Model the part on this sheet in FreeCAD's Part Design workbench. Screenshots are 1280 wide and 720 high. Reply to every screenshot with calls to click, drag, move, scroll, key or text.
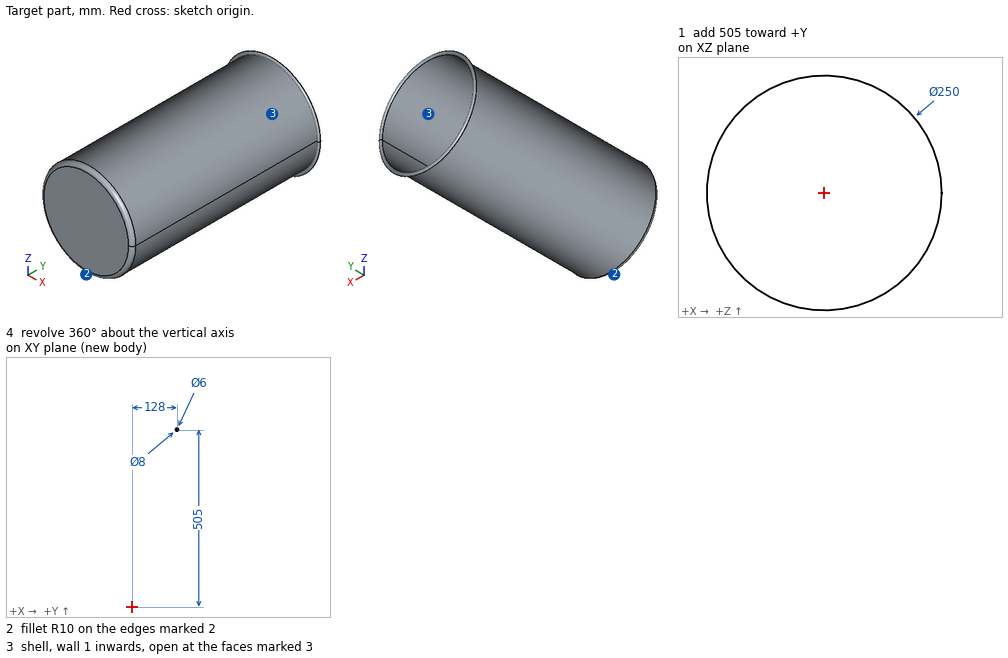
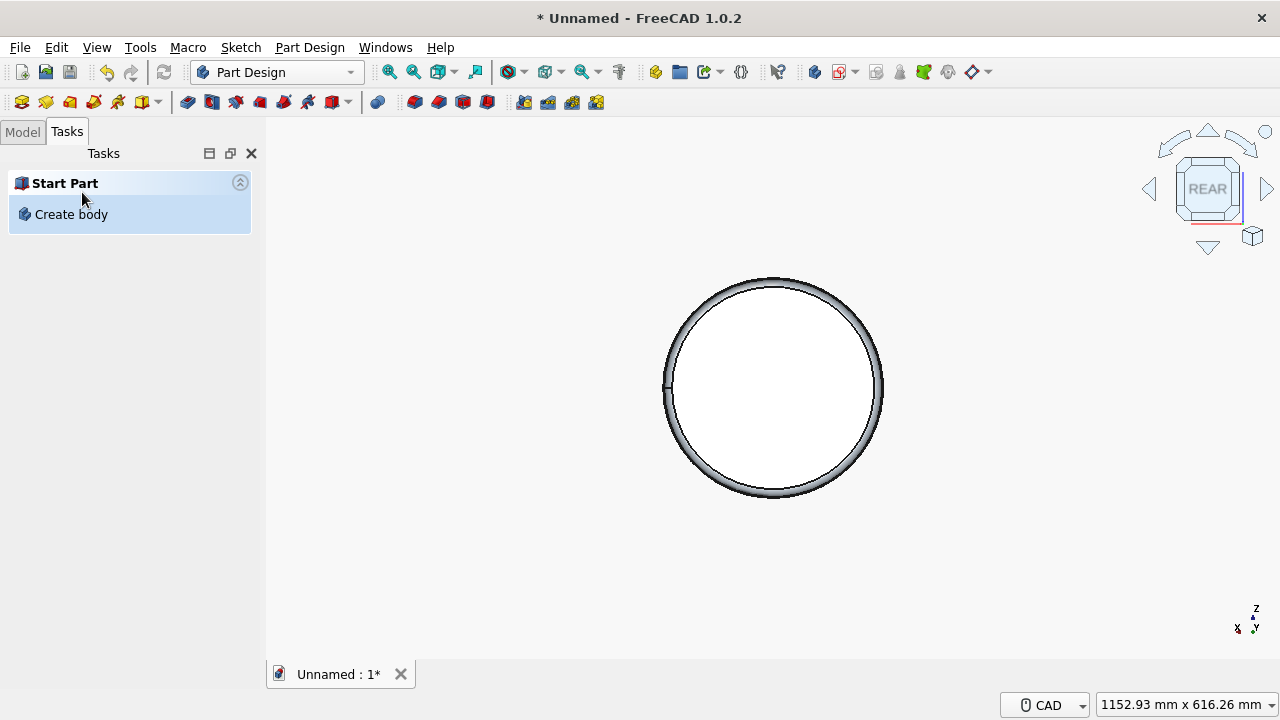
click(390, 72)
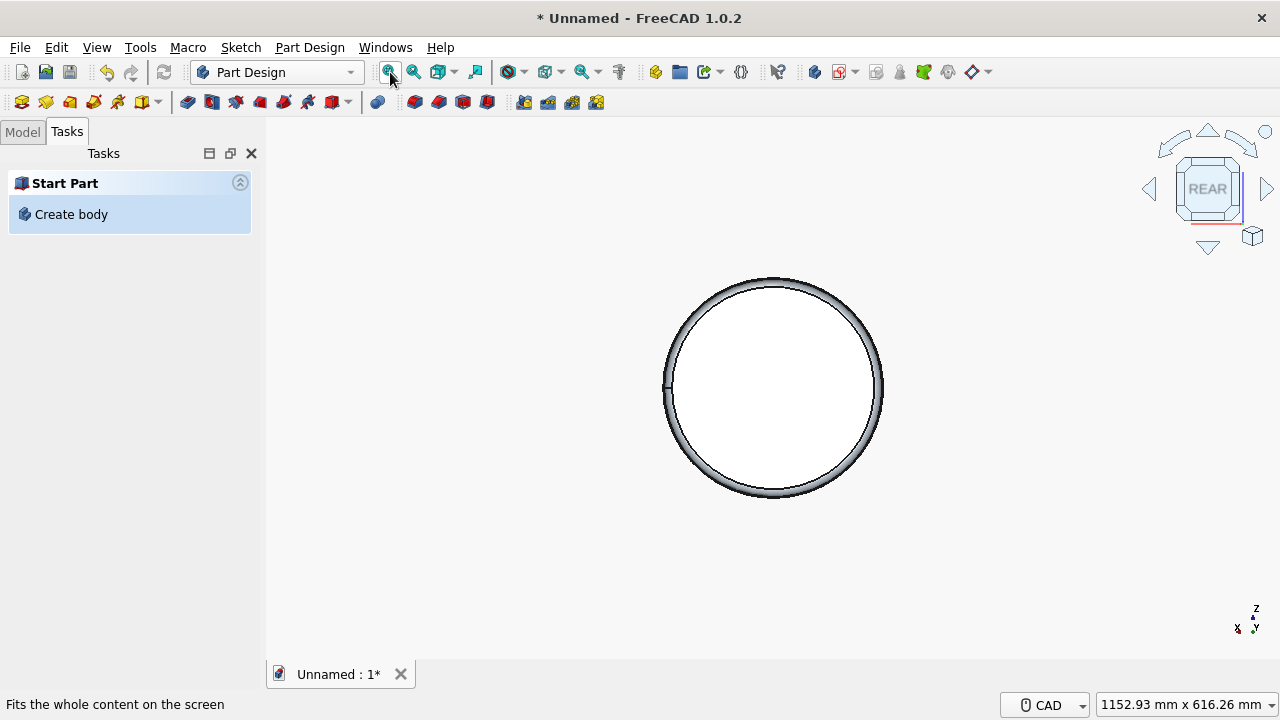
click(816, 72)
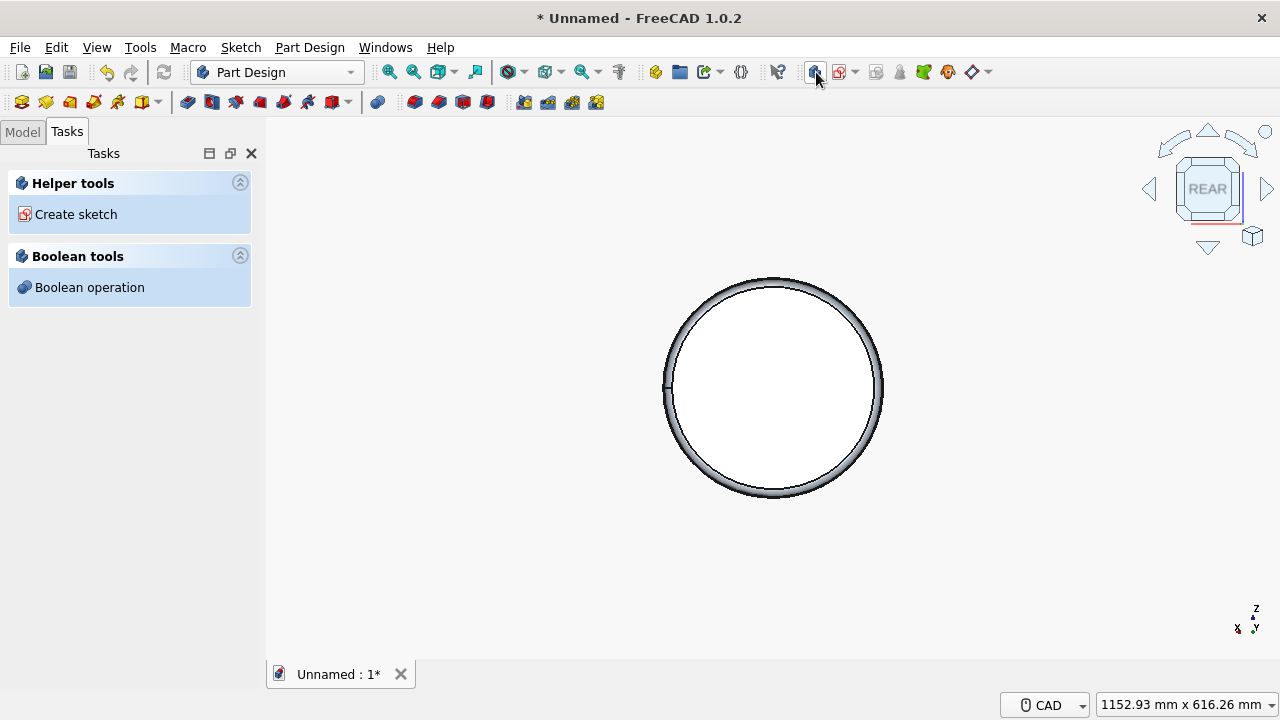
click(306, 619)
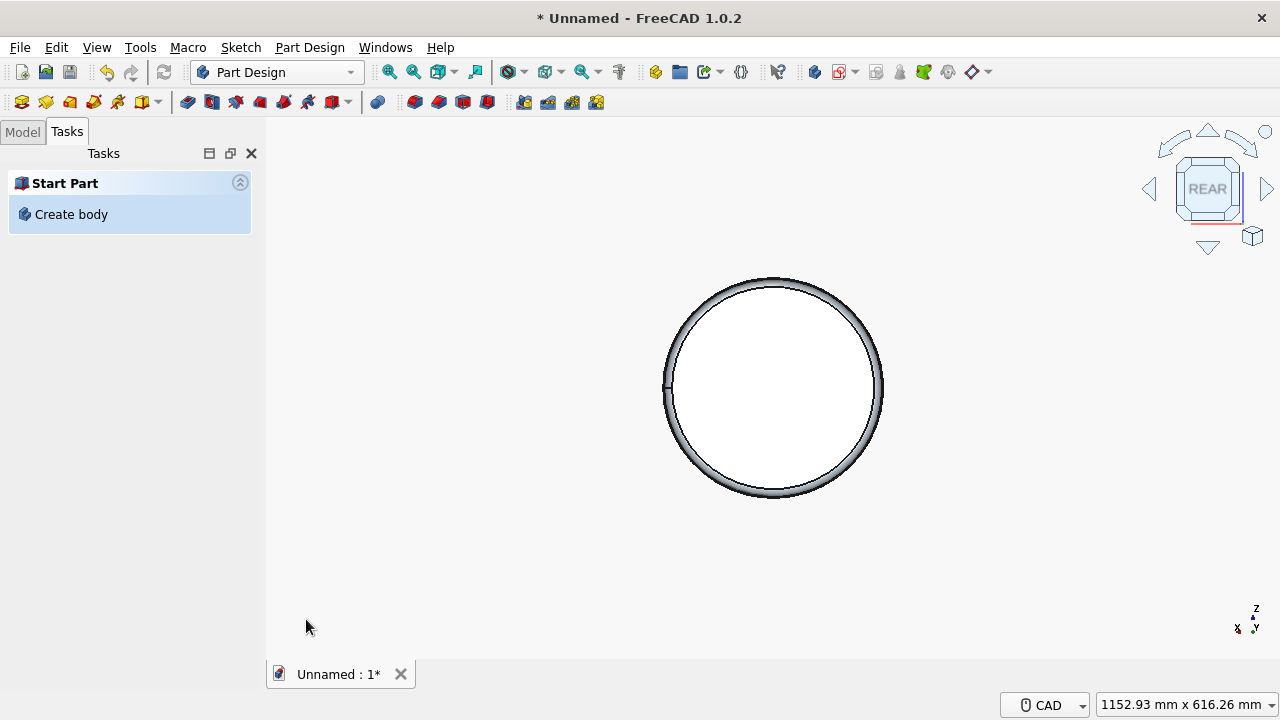
click(840, 72)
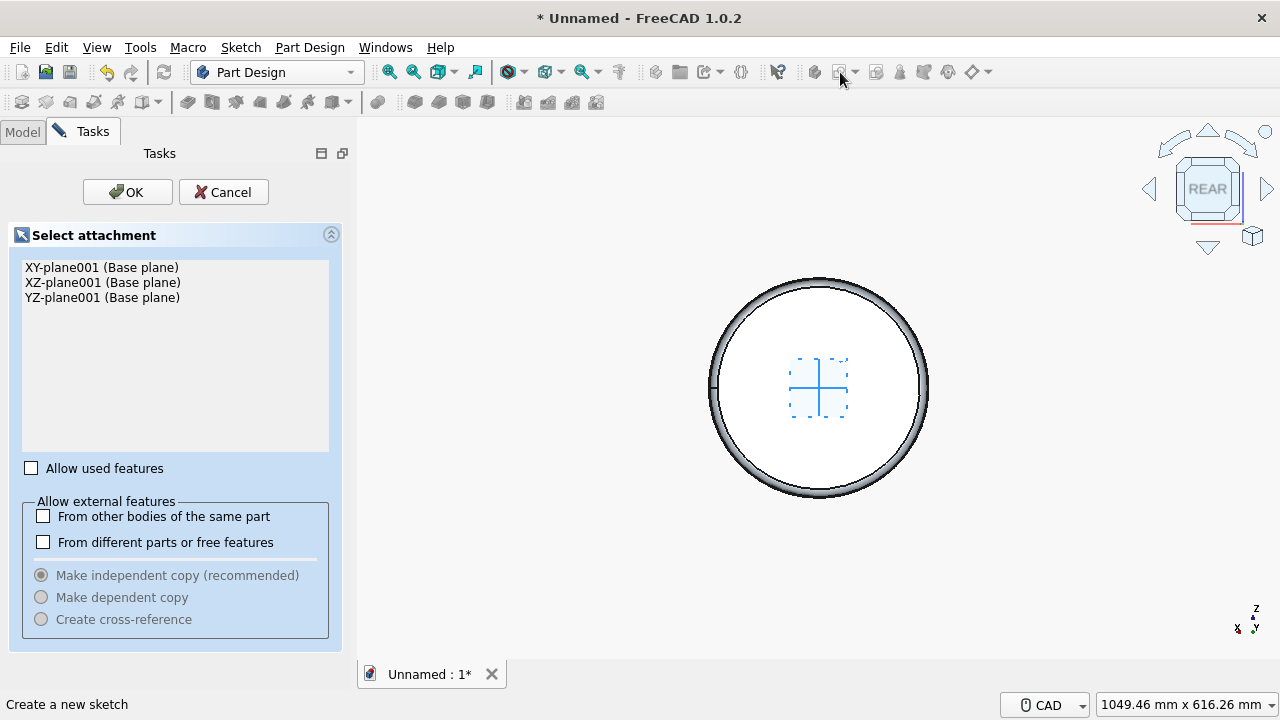
click(82, 268)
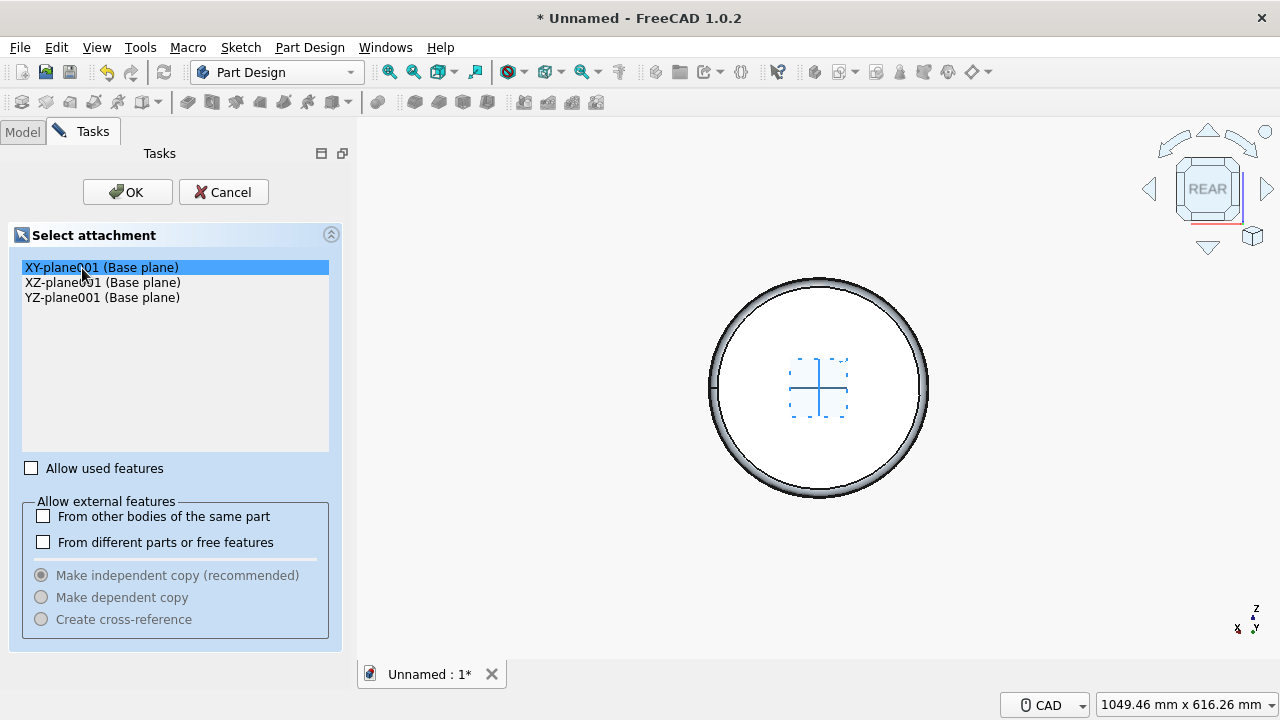
click(128, 192)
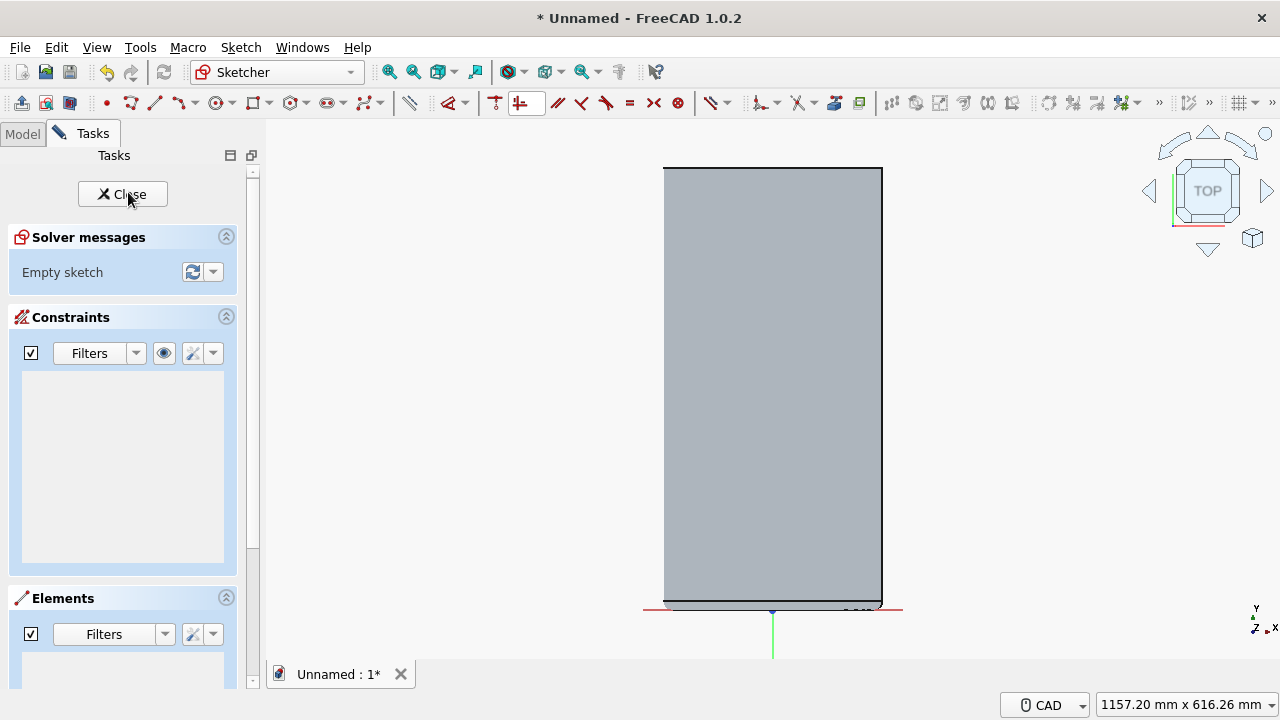
scroll(894, 156, up, 15)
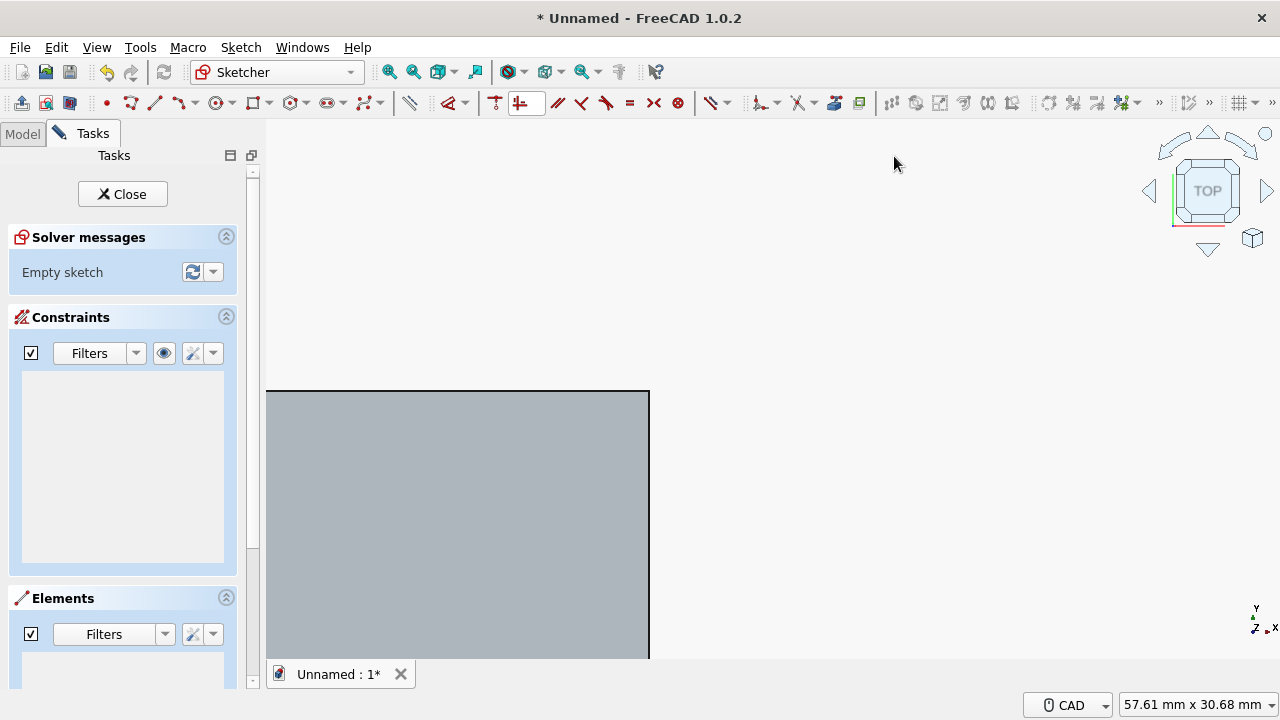
scroll(699, 392, up, 4)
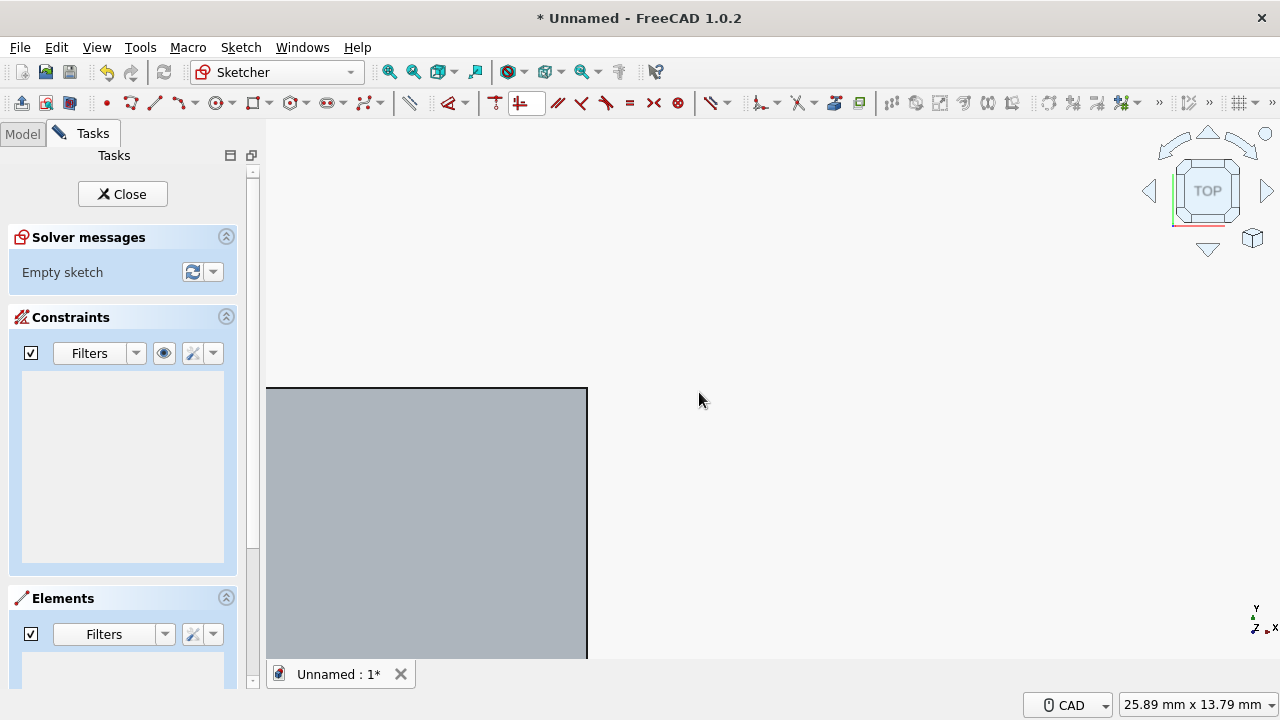
click(216, 104)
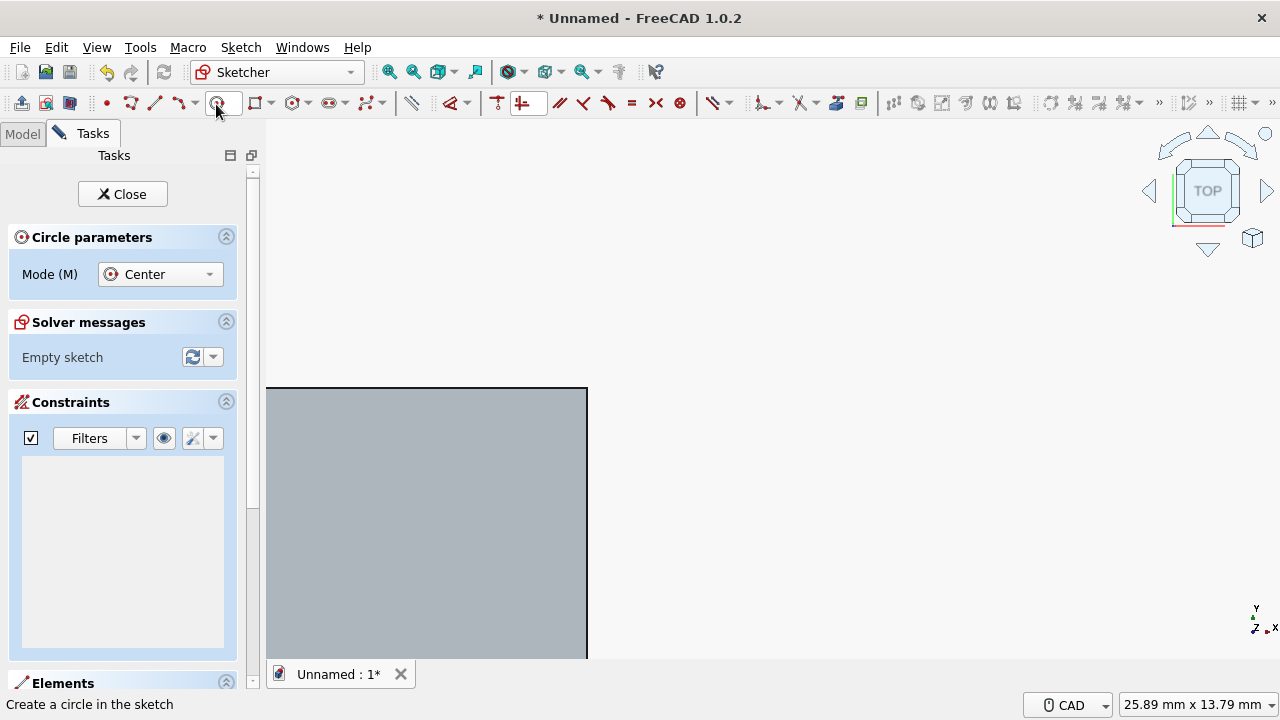
click(704, 388)
move(815, 277)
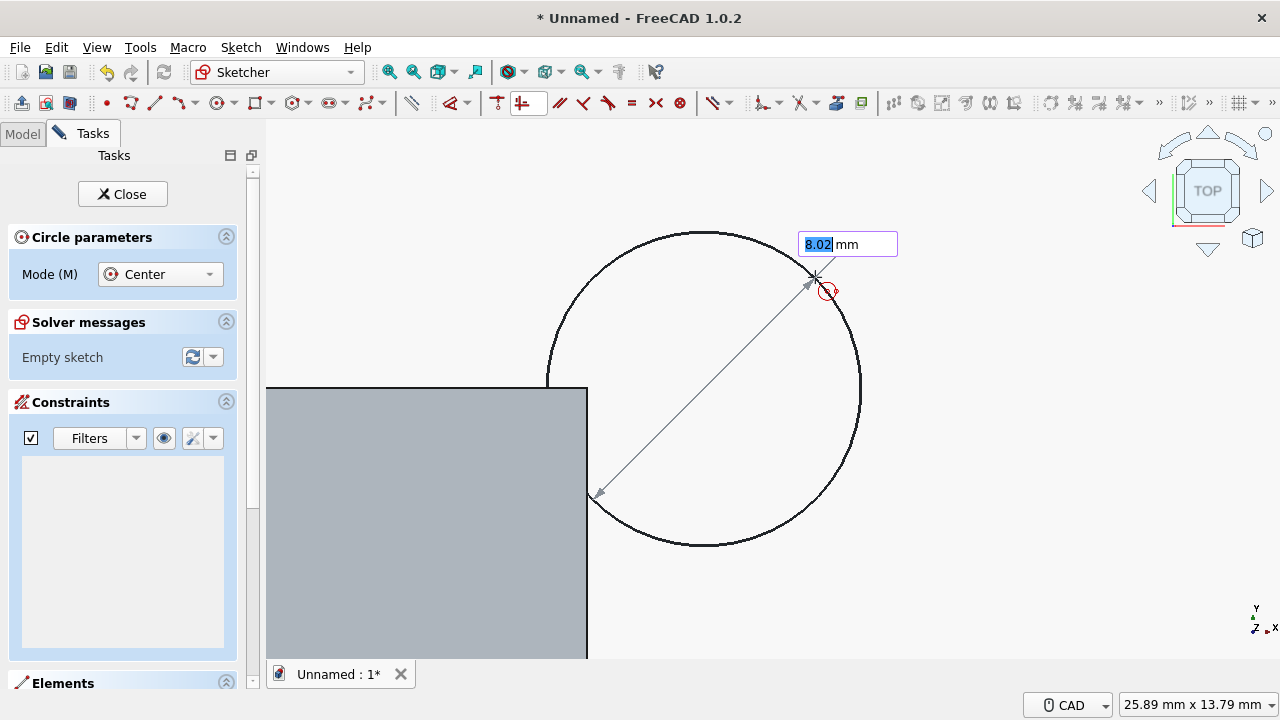
text(8)
key(Return)